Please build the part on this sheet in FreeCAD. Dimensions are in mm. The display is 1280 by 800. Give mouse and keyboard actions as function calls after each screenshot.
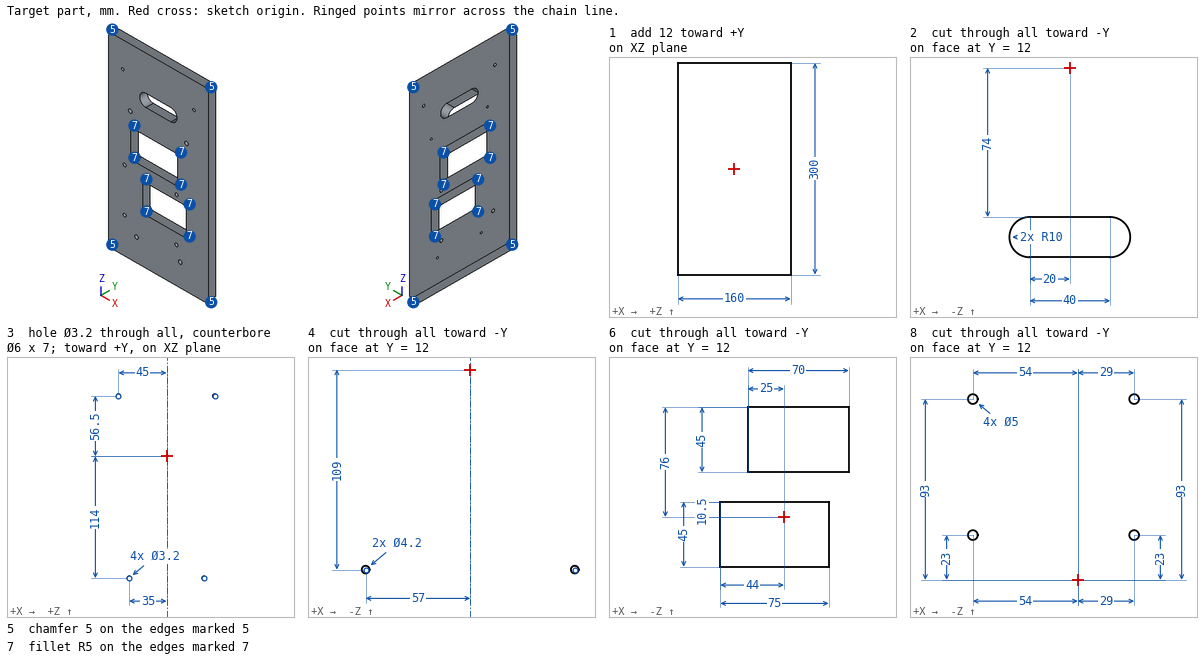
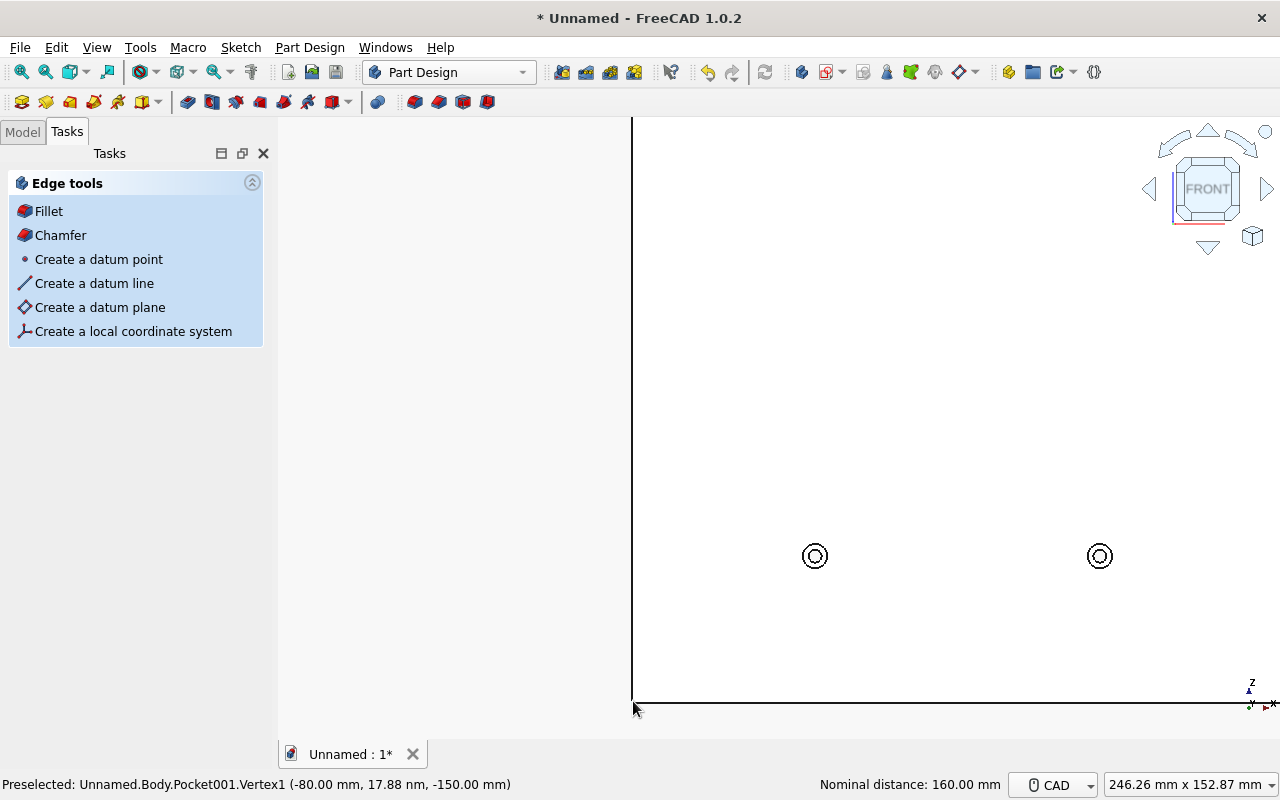
click(22, 72)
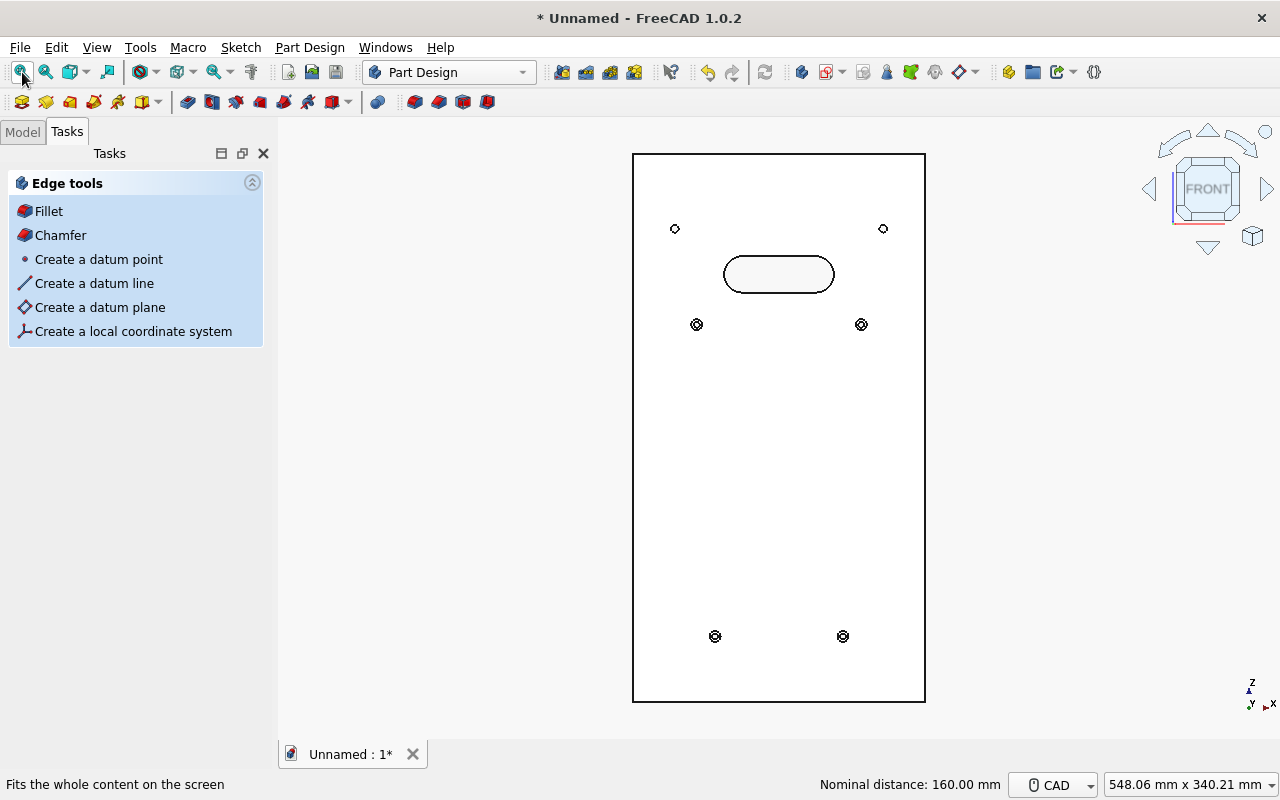
key(3)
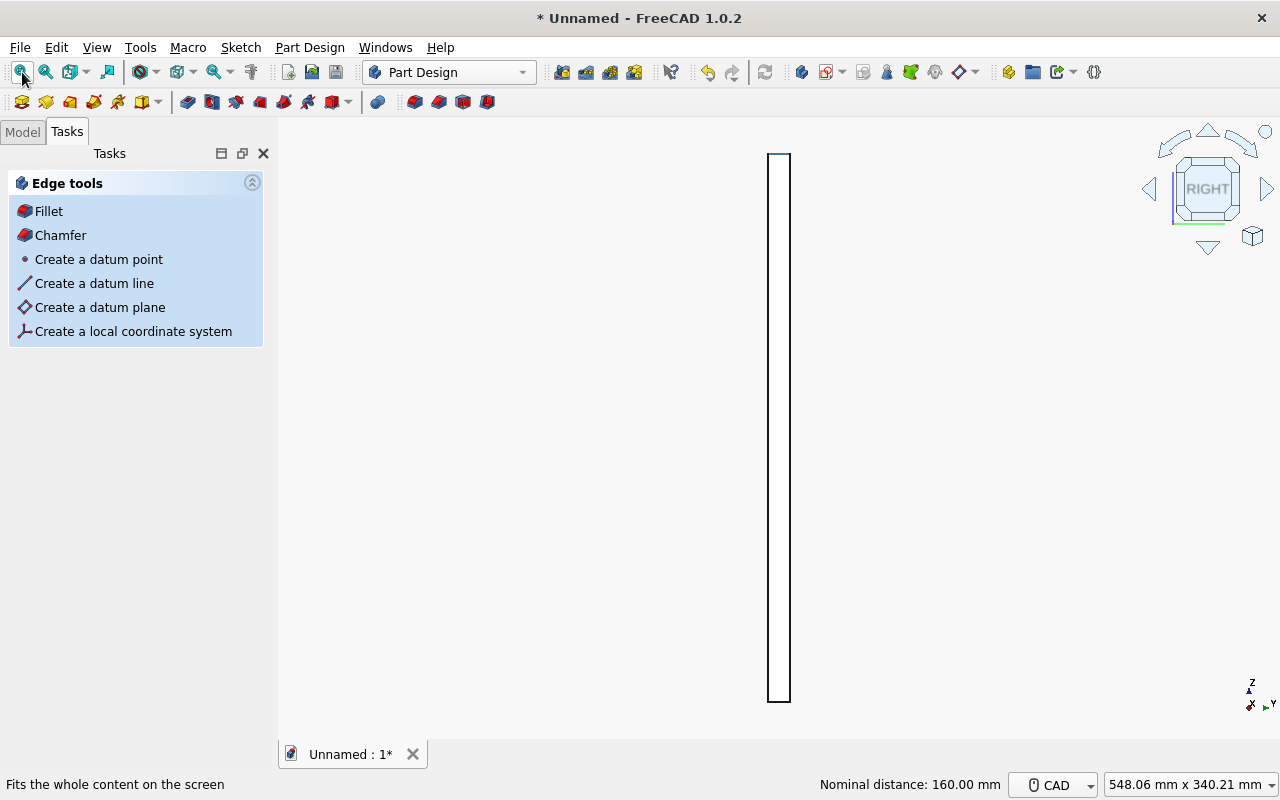
click(779, 701, ctrl)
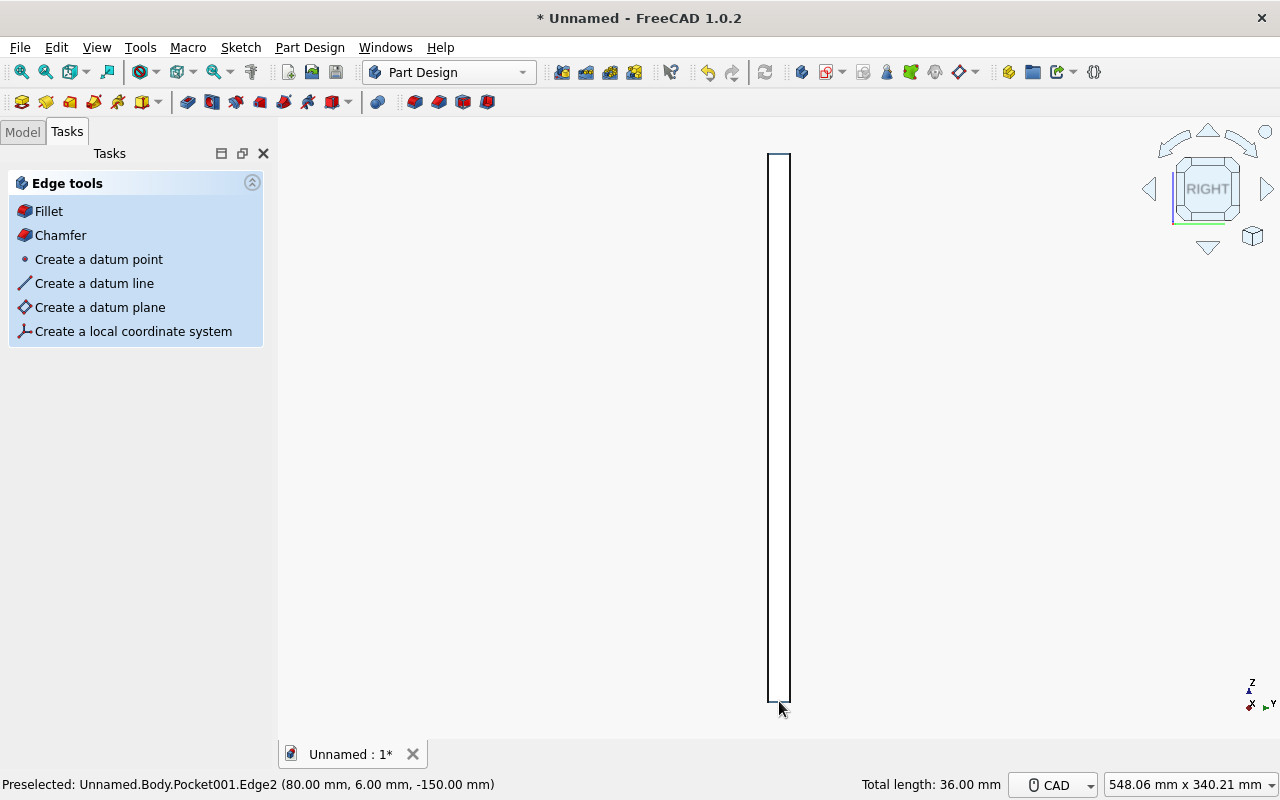
scroll(779, 701, up, 4)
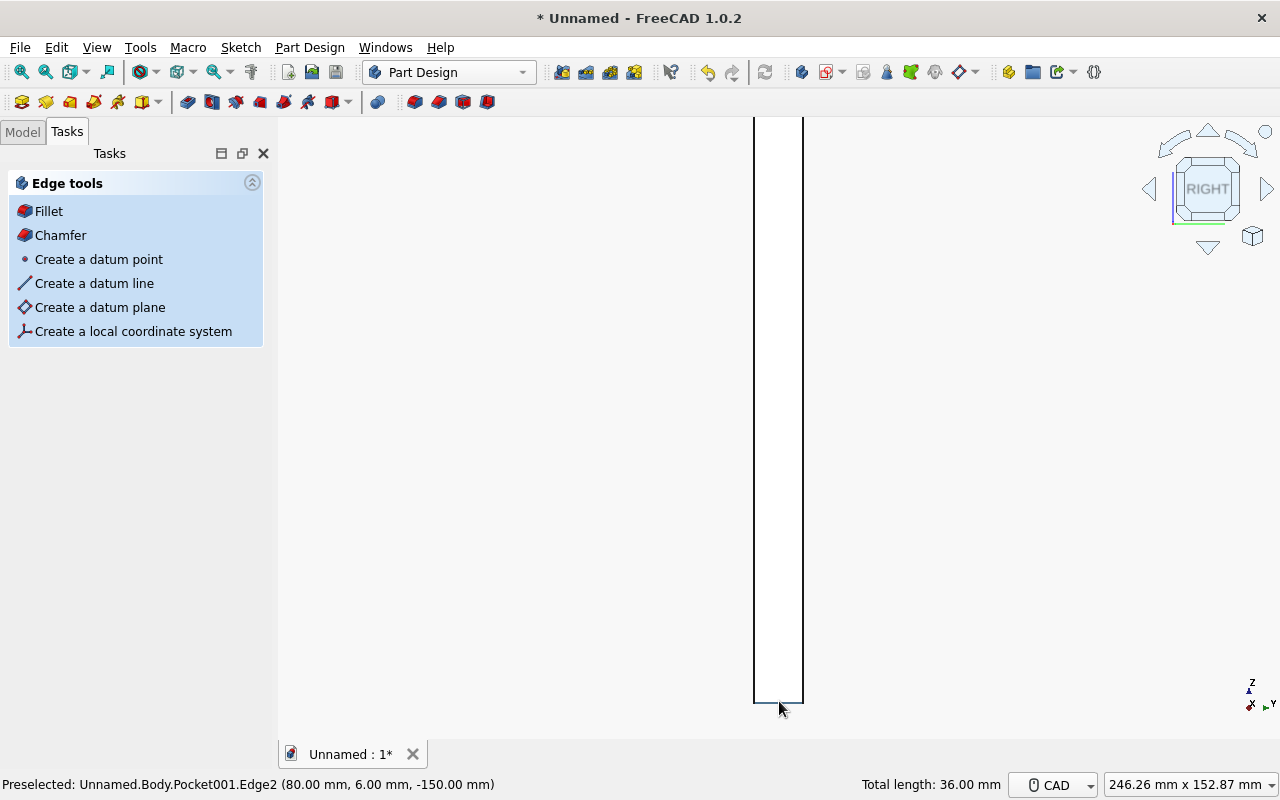
click(22, 72)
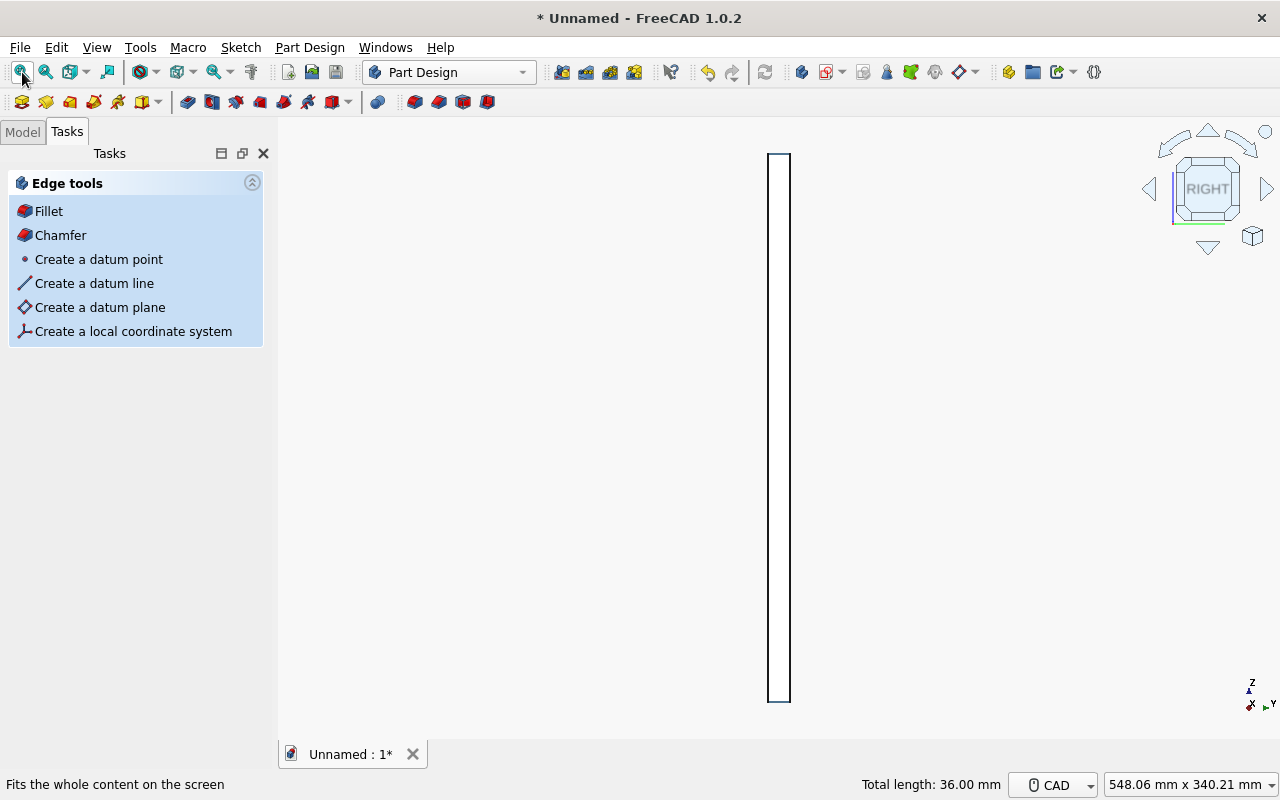
key(5)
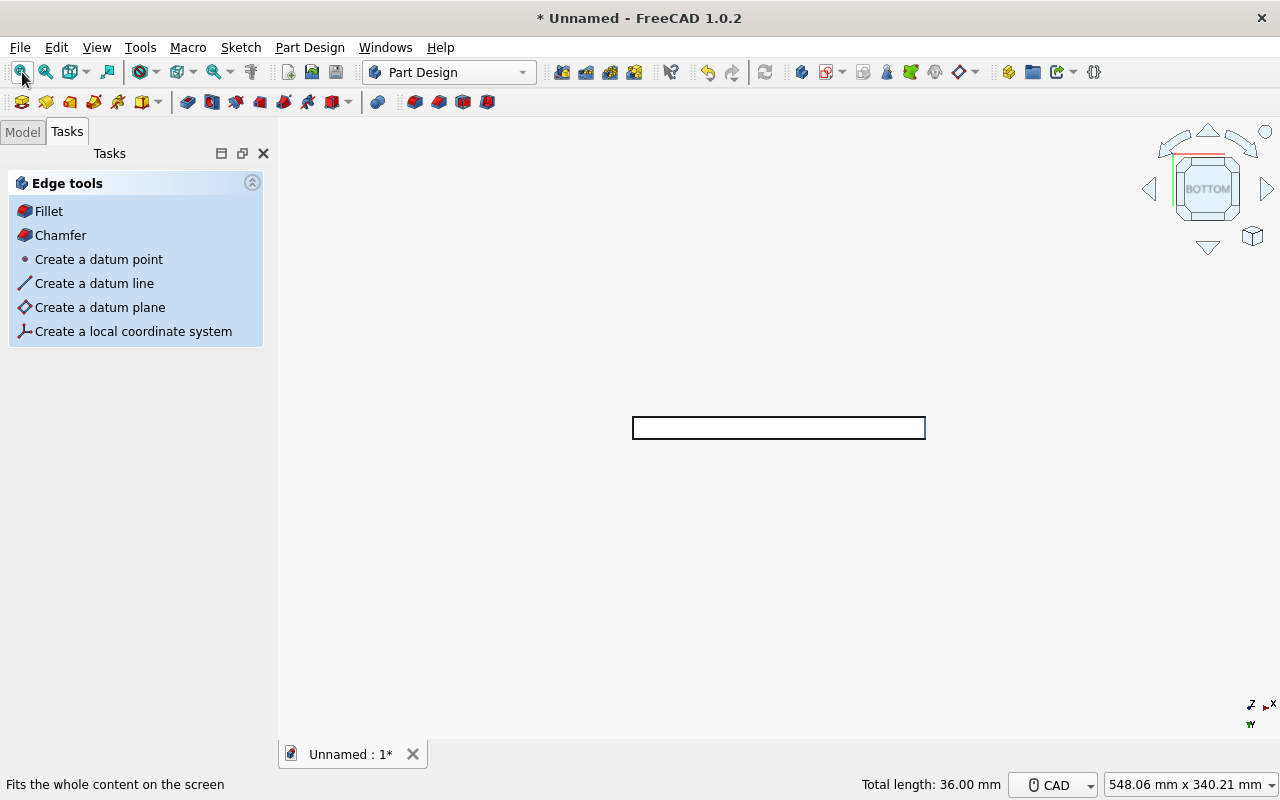
click(22, 72)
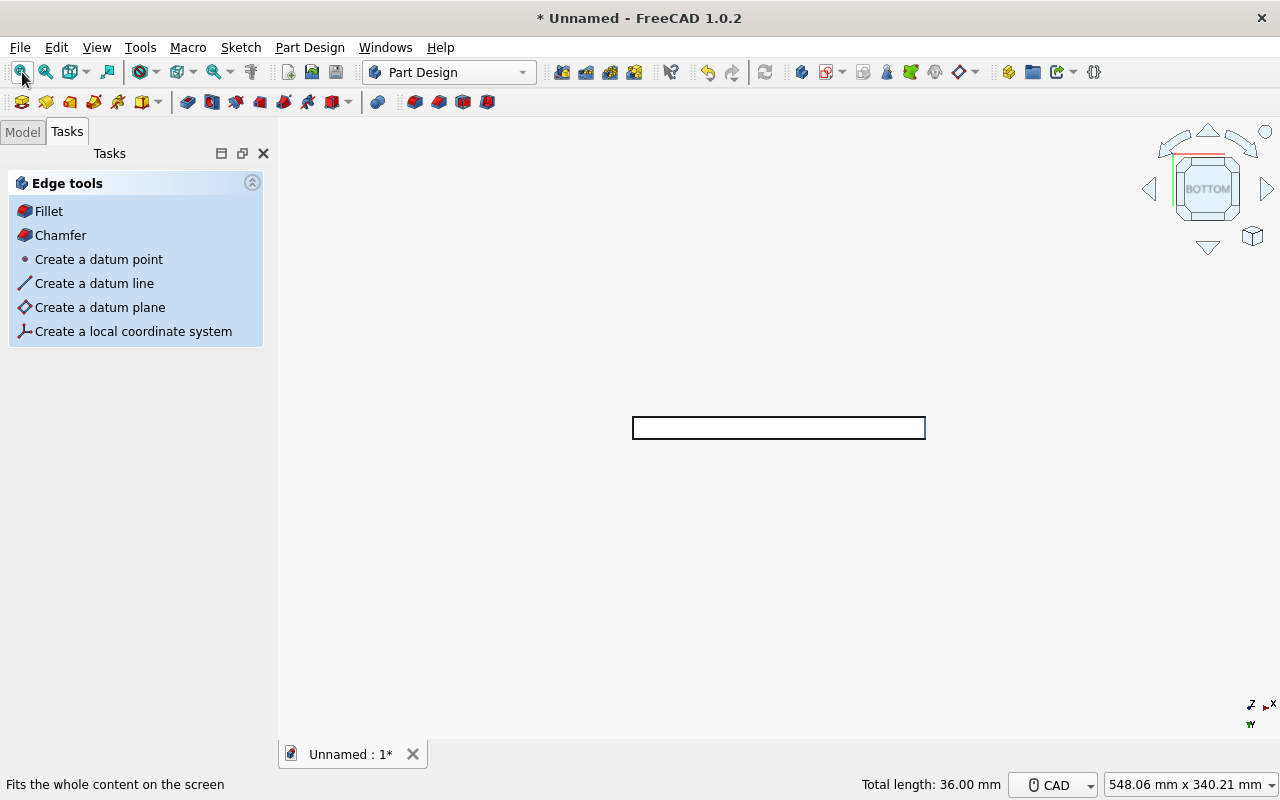
click(633, 427, ctrl)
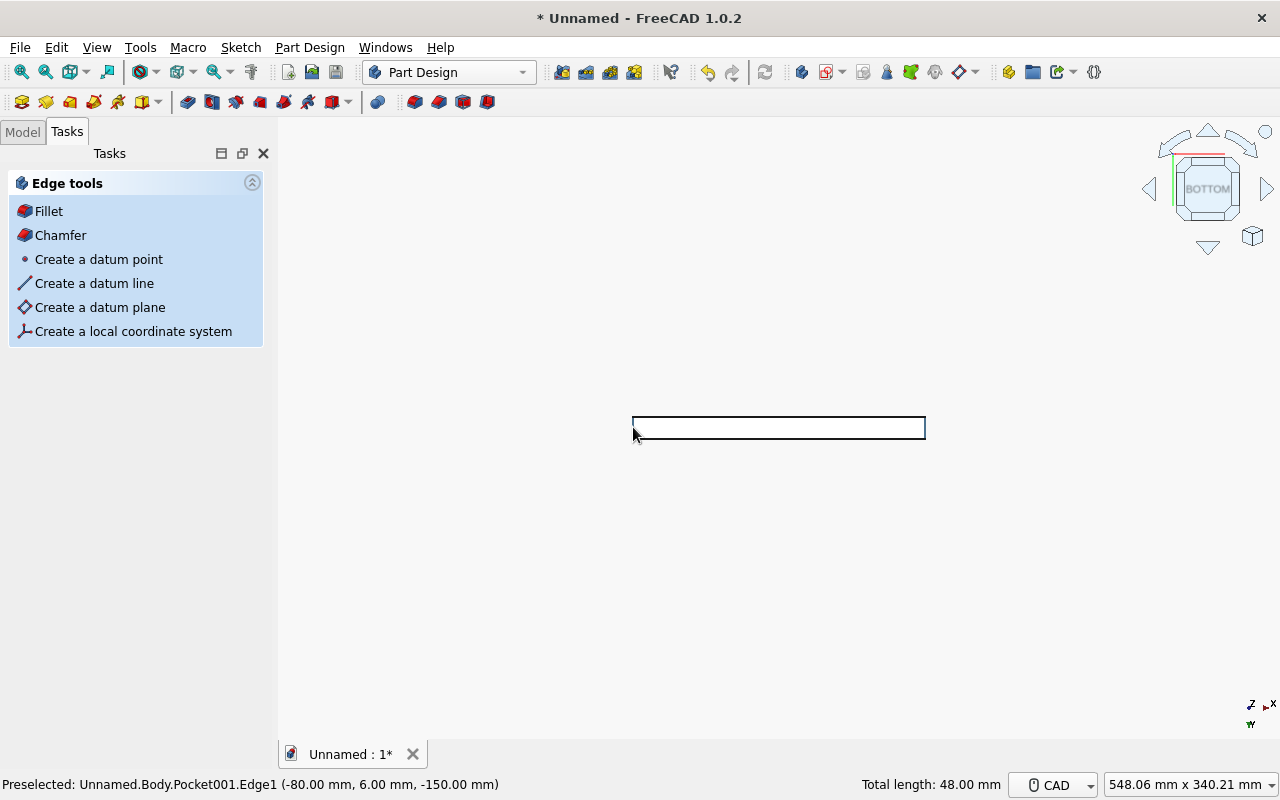
click(440, 102)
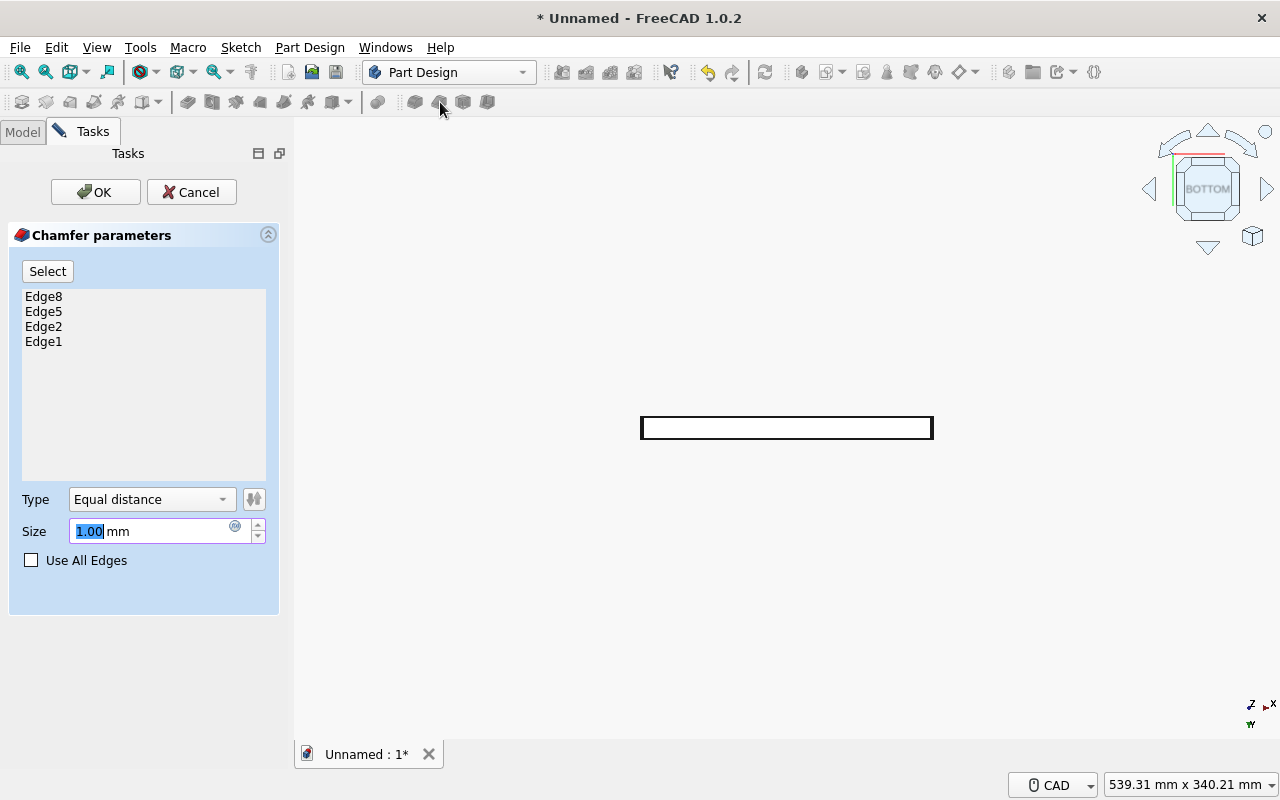
text(5)
key(Tab)